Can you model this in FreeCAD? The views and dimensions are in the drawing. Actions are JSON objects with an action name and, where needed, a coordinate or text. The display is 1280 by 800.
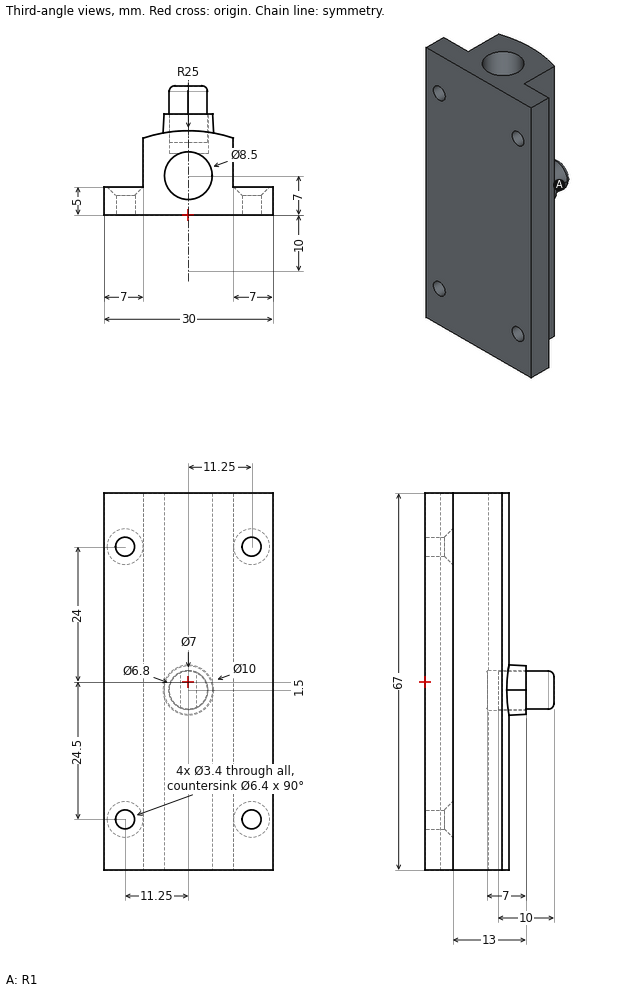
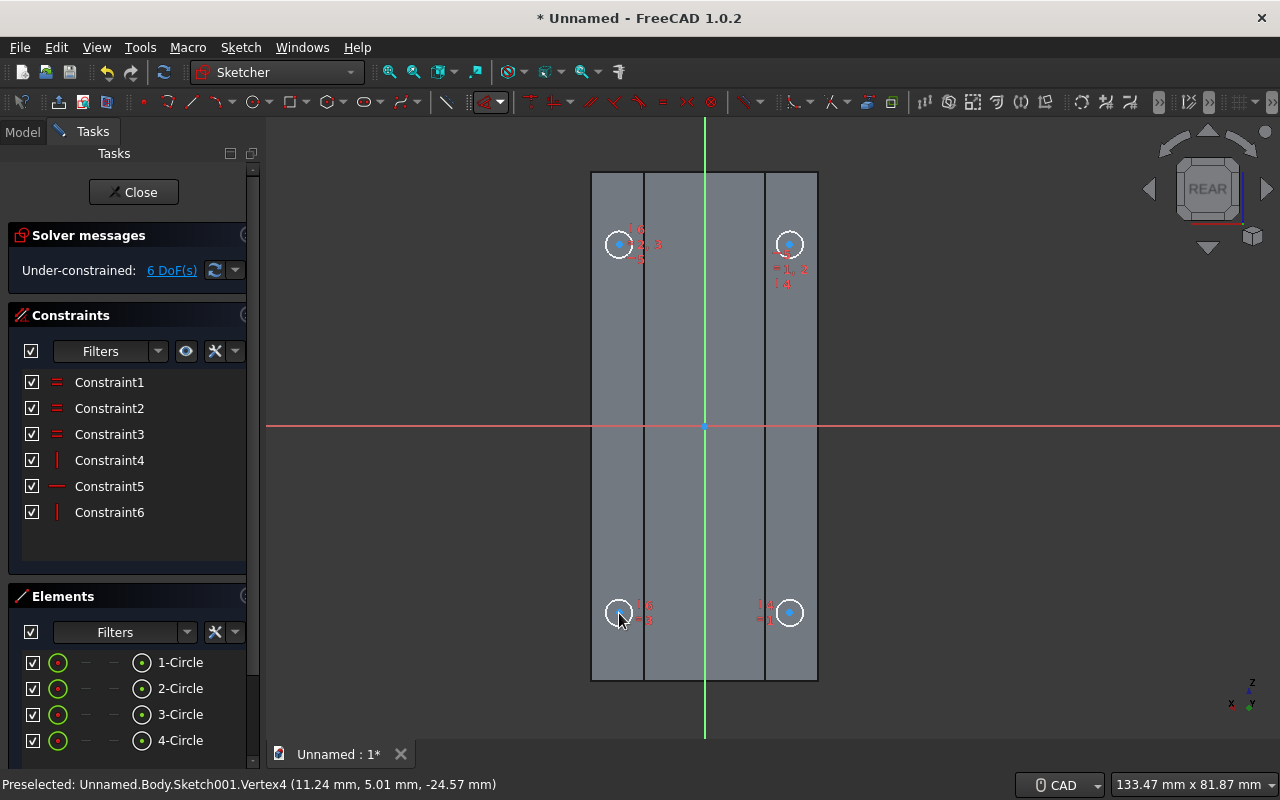
{"action": "left_click", "coordinate": [790, 613]}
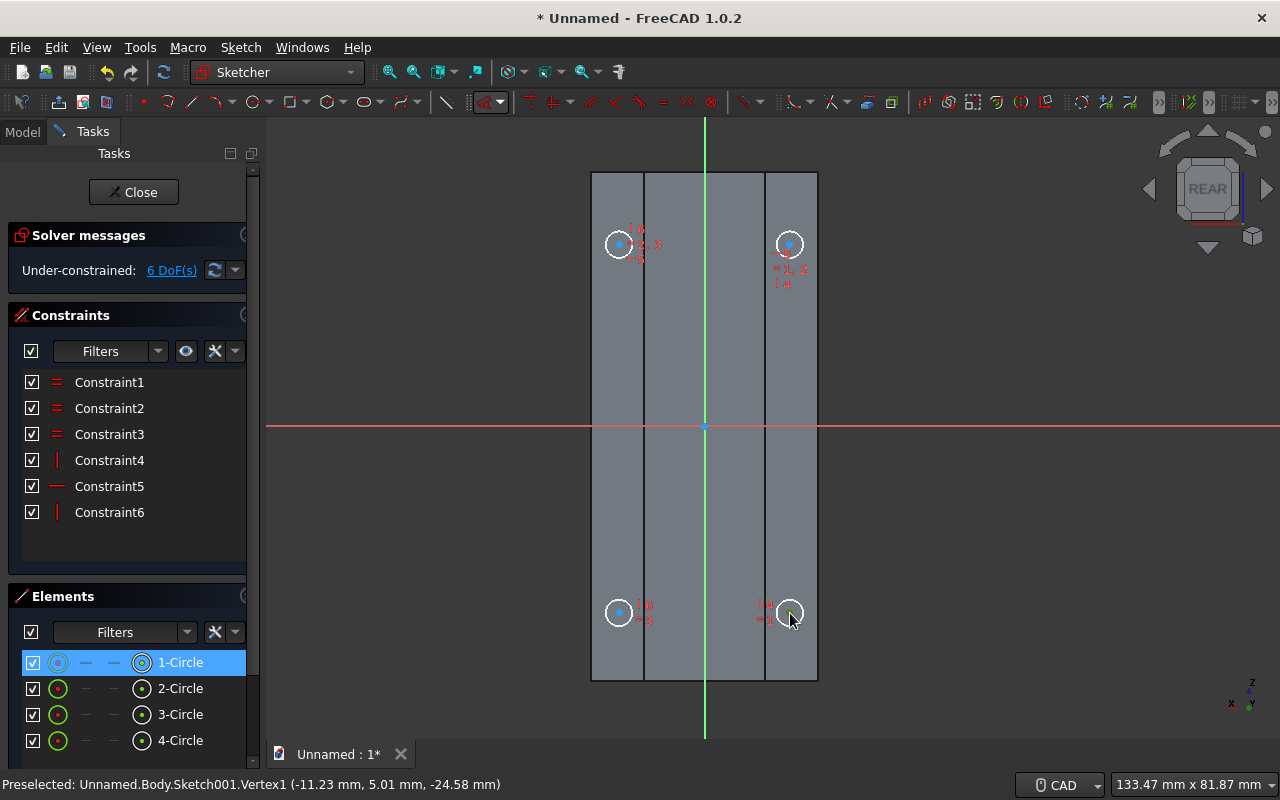
{"action": "left_click", "coordinate": [619, 613]}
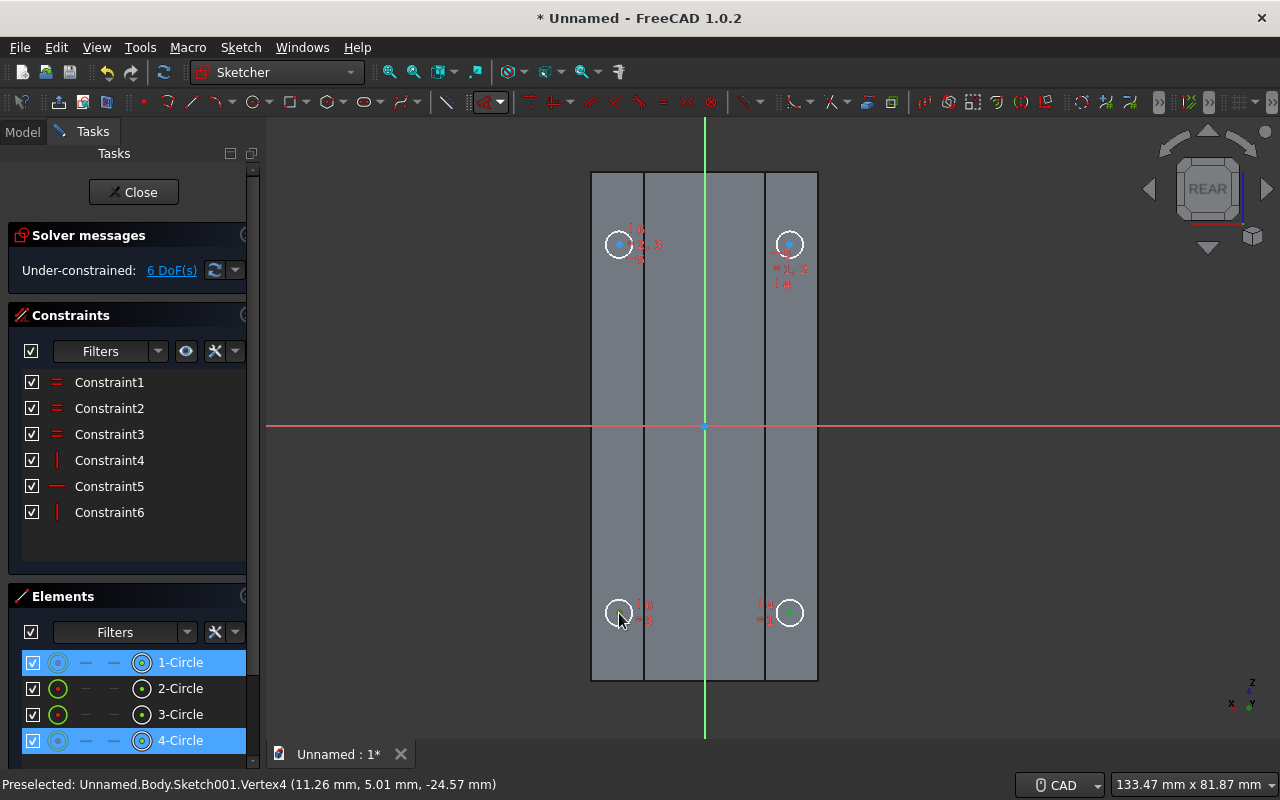
{"action": "key", "text": "h"}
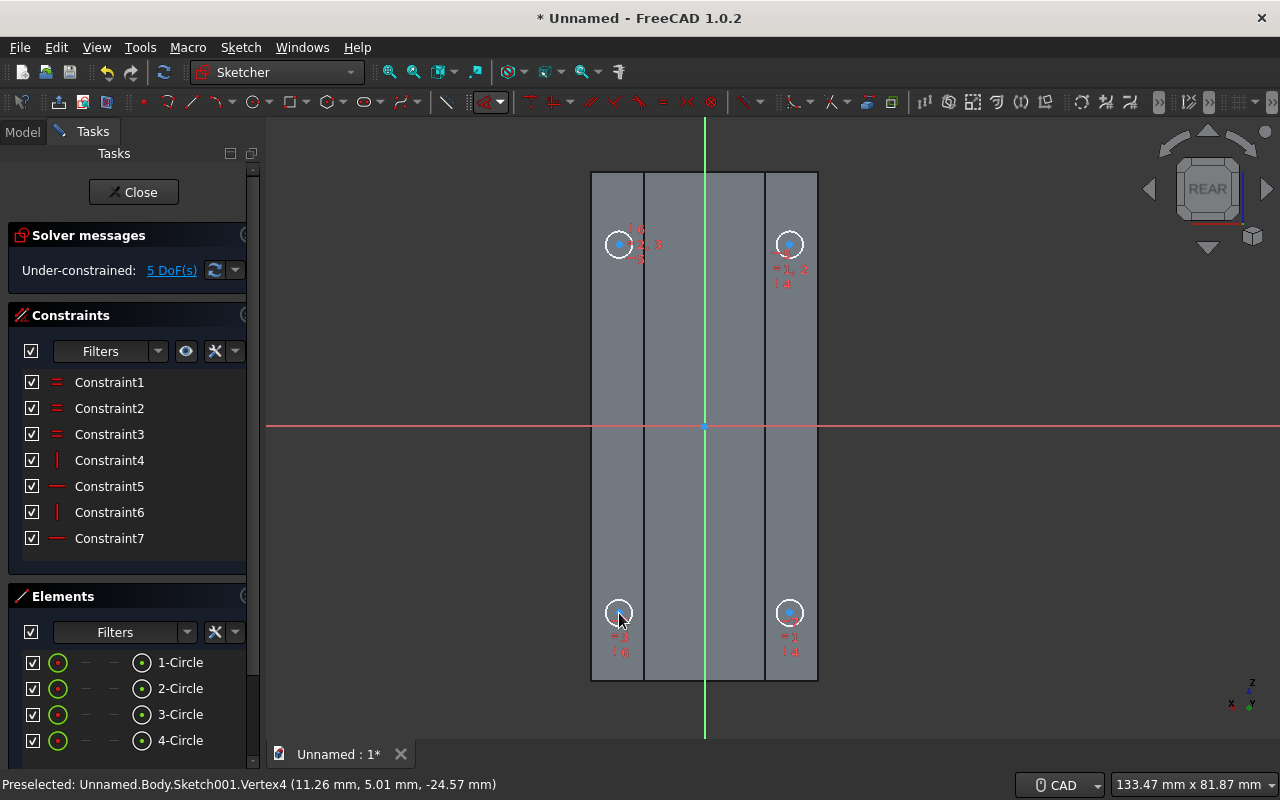
{"action": "scroll", "coordinate": [799, 604], "scroll_direction": "up", "scroll_amount": 3}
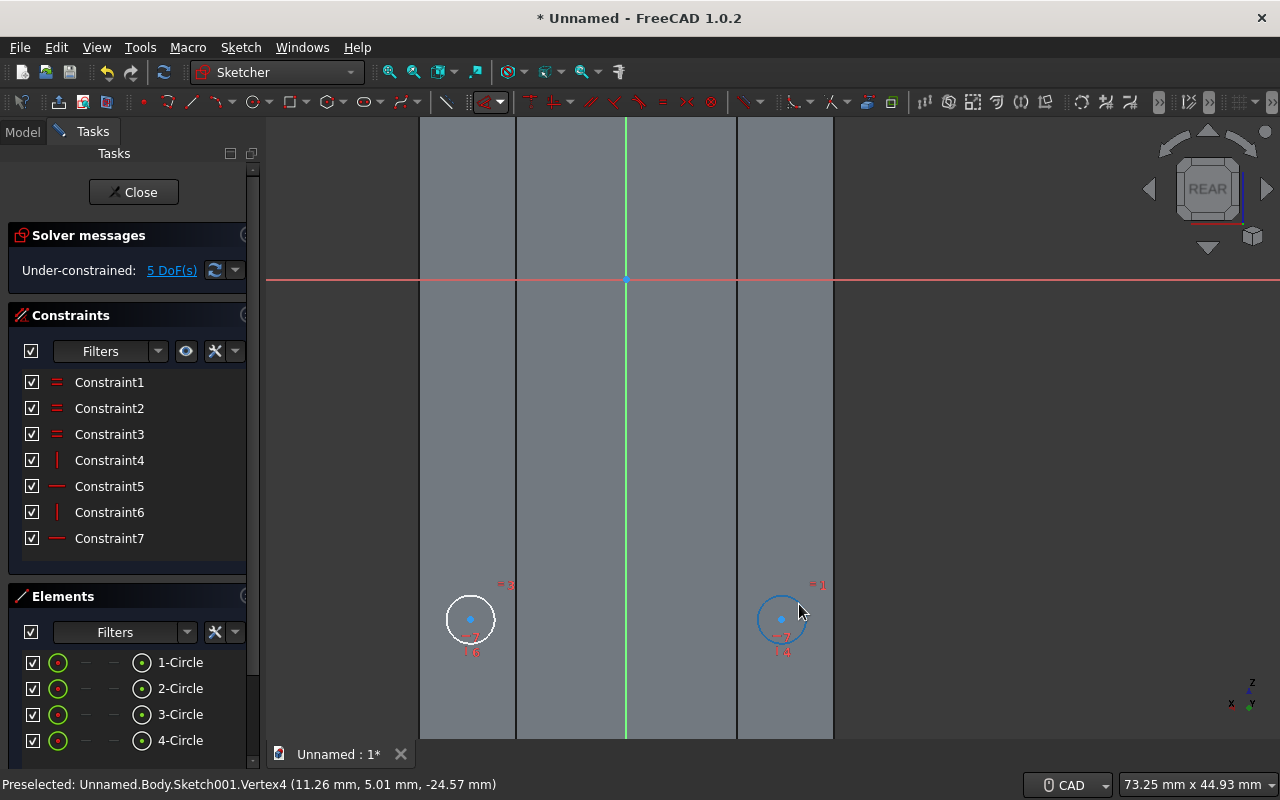
{"action": "left_click", "coordinate": [799, 603]}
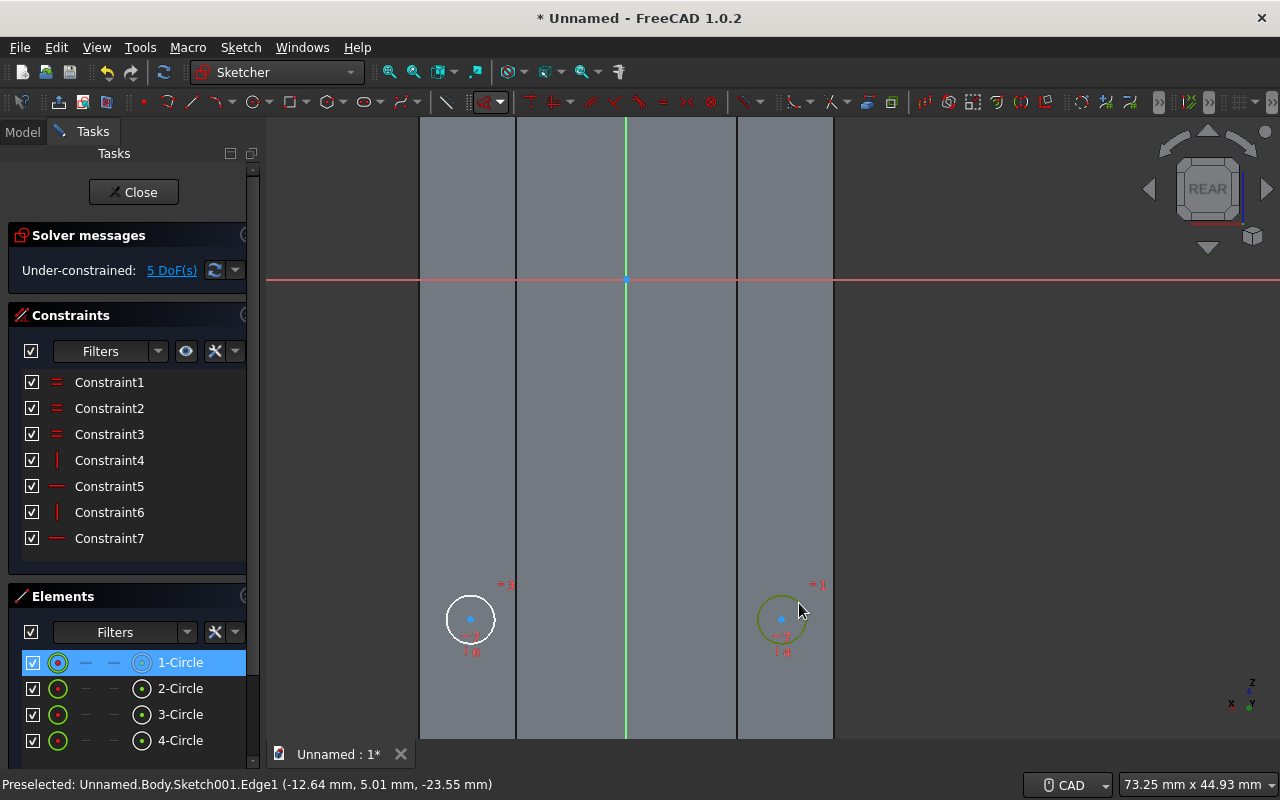
{"action": "key", "text": "k o"}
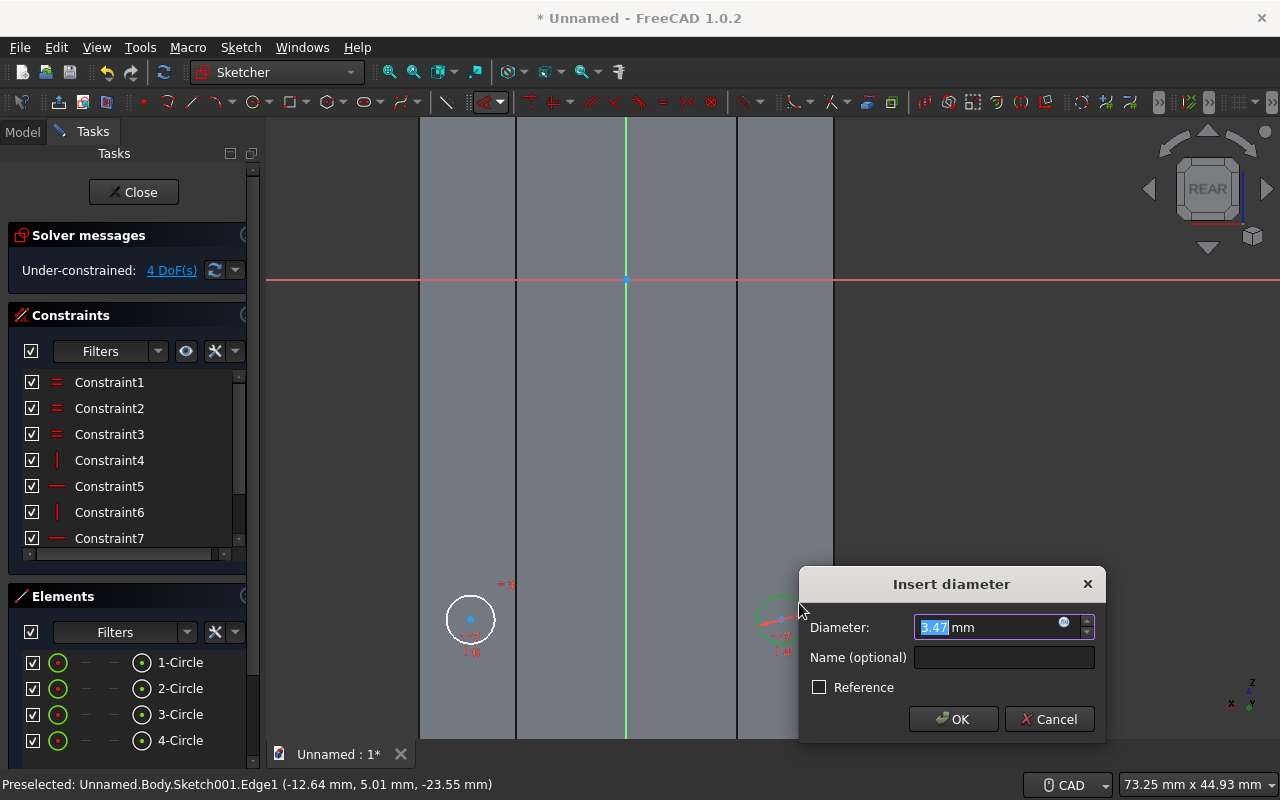
{"action": "type", "text": "3.4"}
{"action": "key", "text": "Return"}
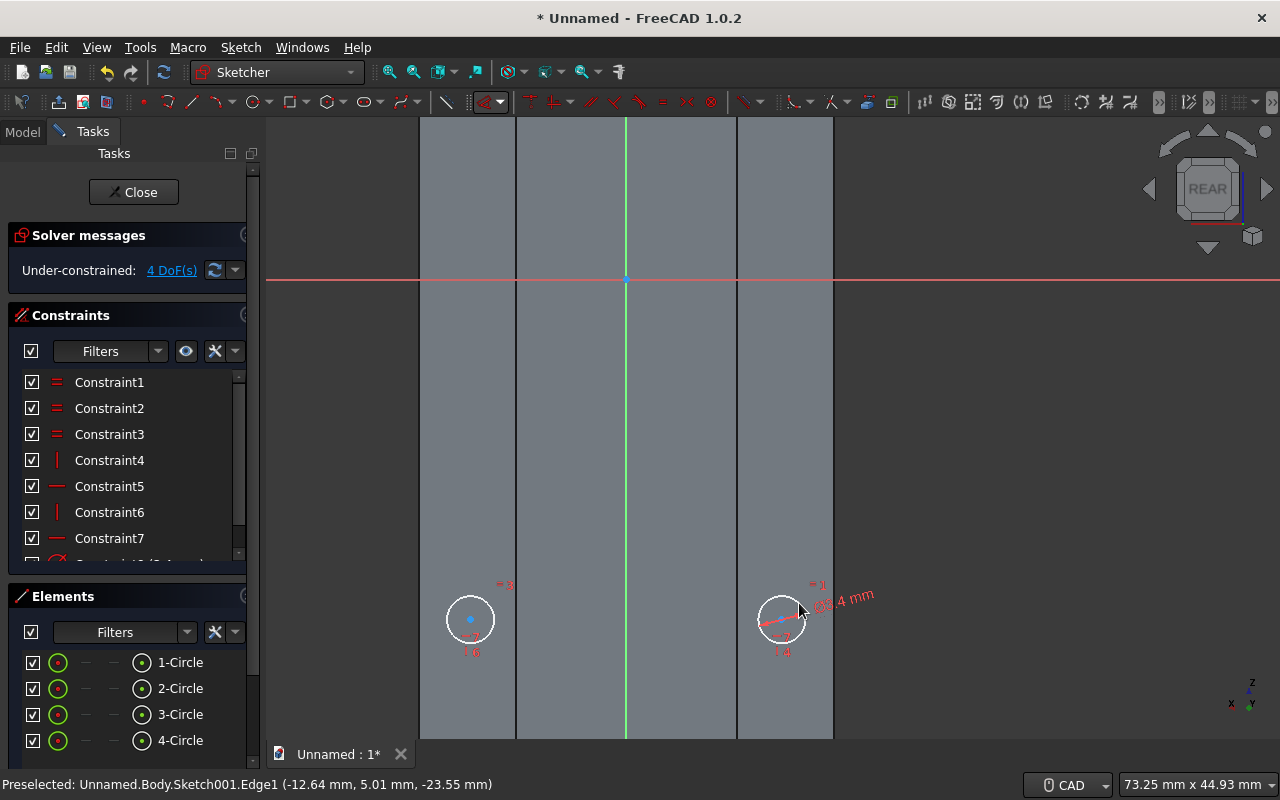
{"action": "scroll", "coordinate": [799, 604], "scroll_direction": "down", "scroll_amount": 3}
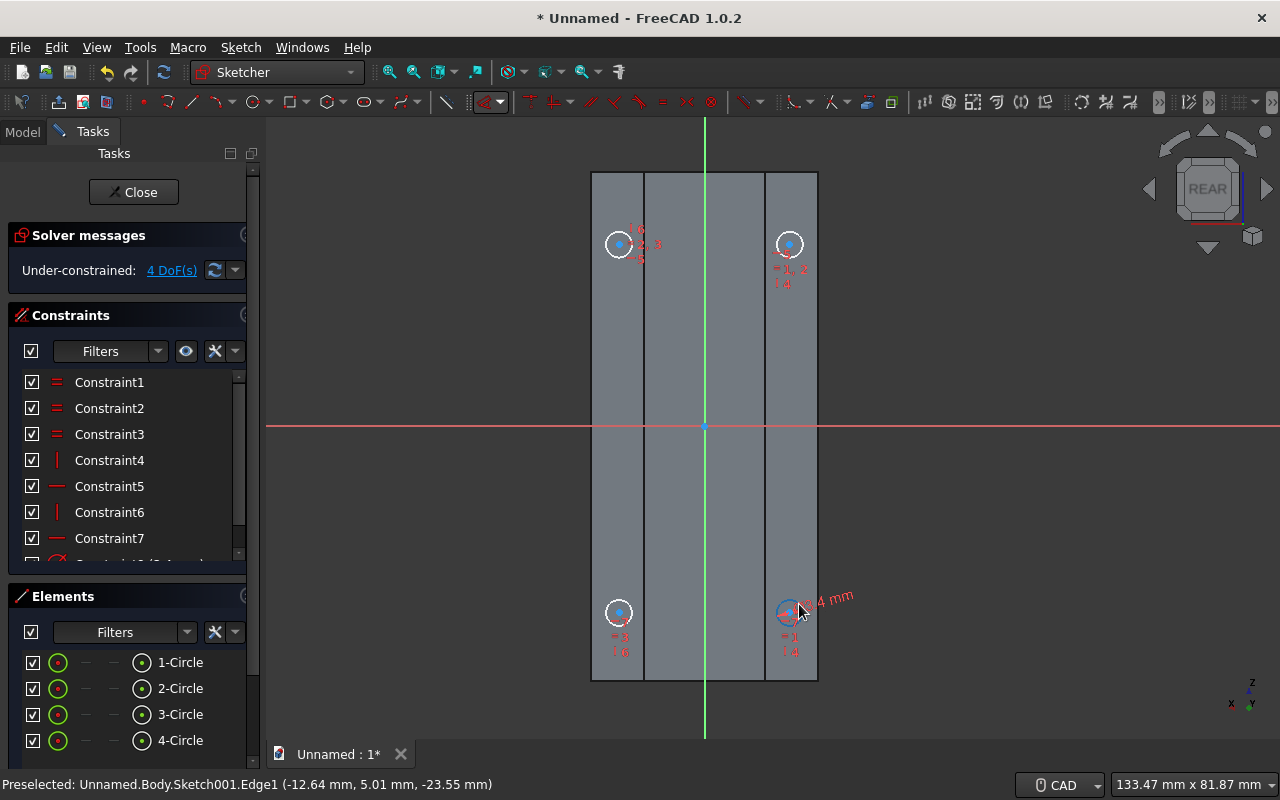
{"action": "left_click", "coordinate": [790, 245]}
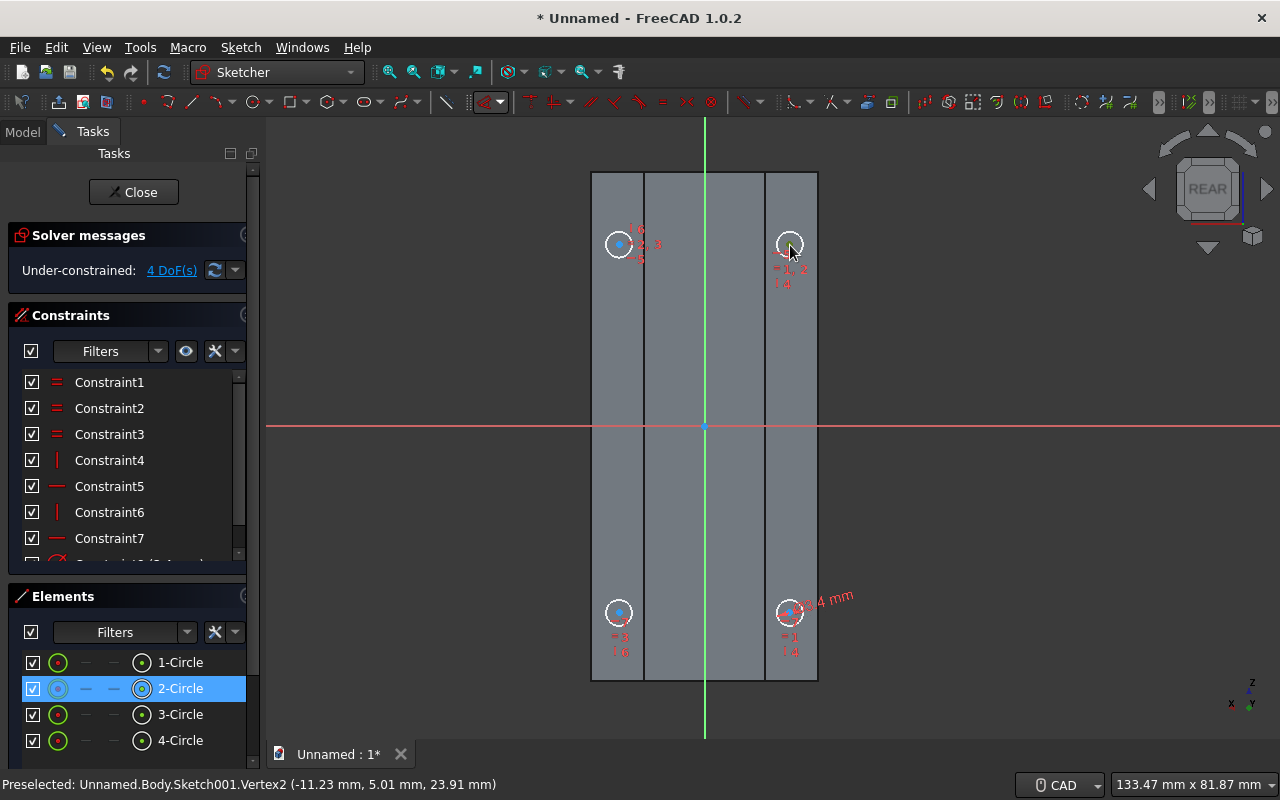
{"action": "key", "text": "i"}